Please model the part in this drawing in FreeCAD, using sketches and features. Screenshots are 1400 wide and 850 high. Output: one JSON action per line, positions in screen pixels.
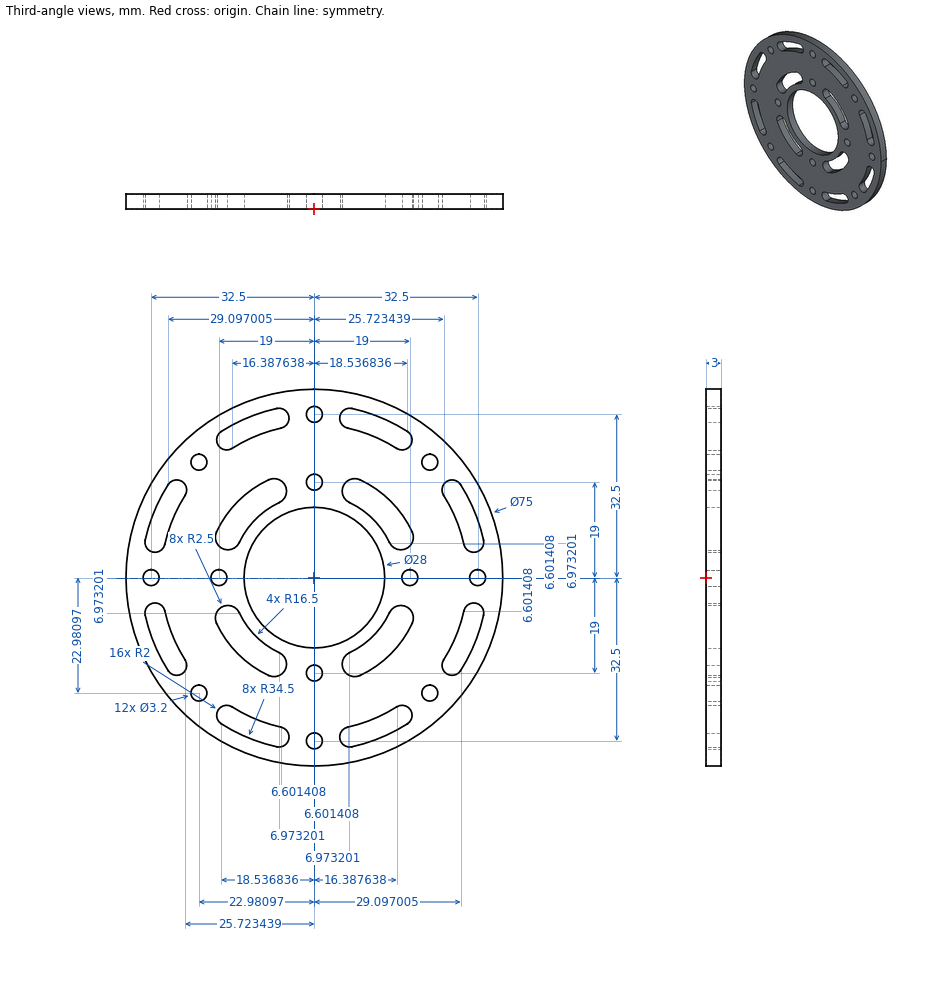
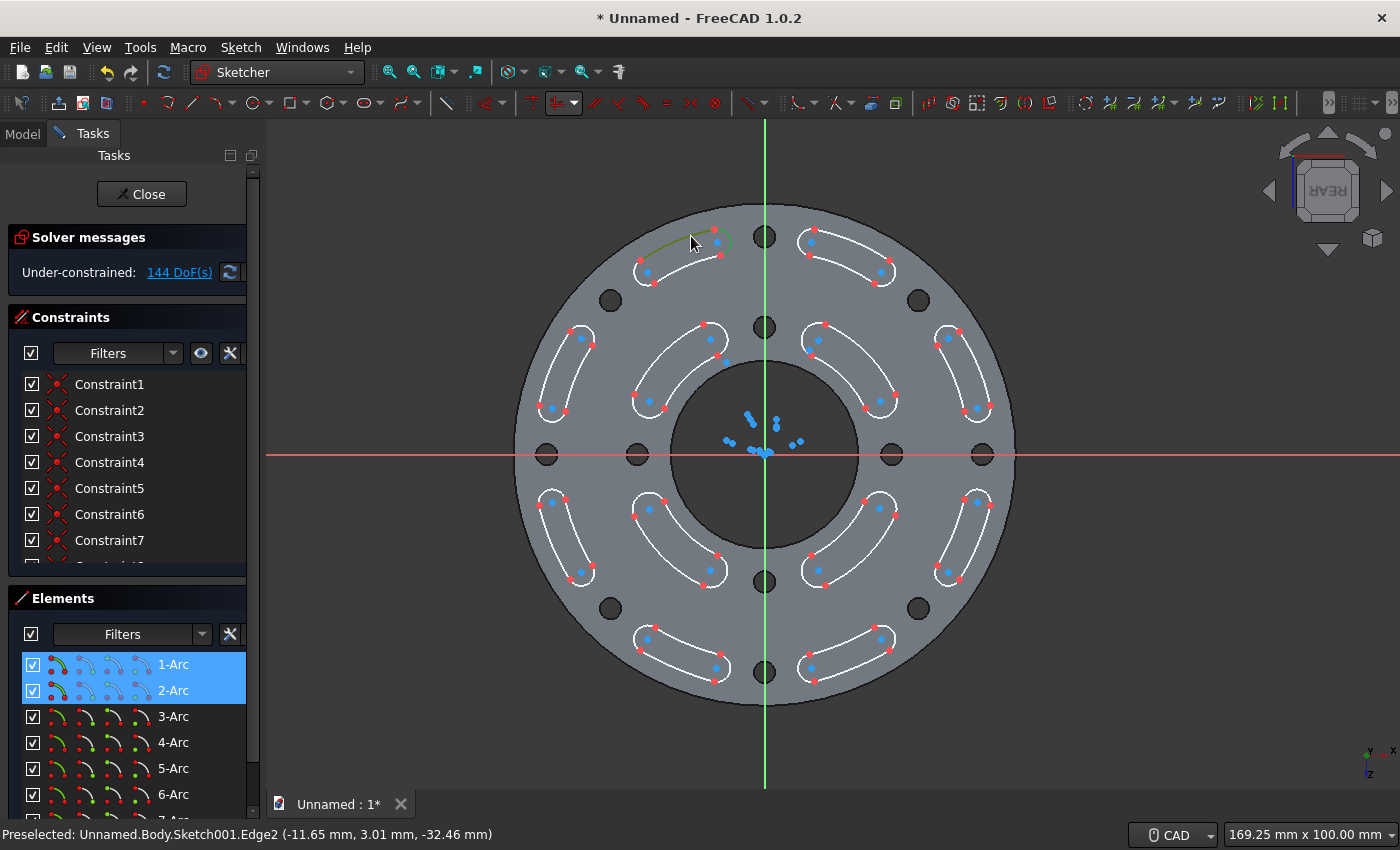
{"action": "left_click", "coordinate": [644, 104]}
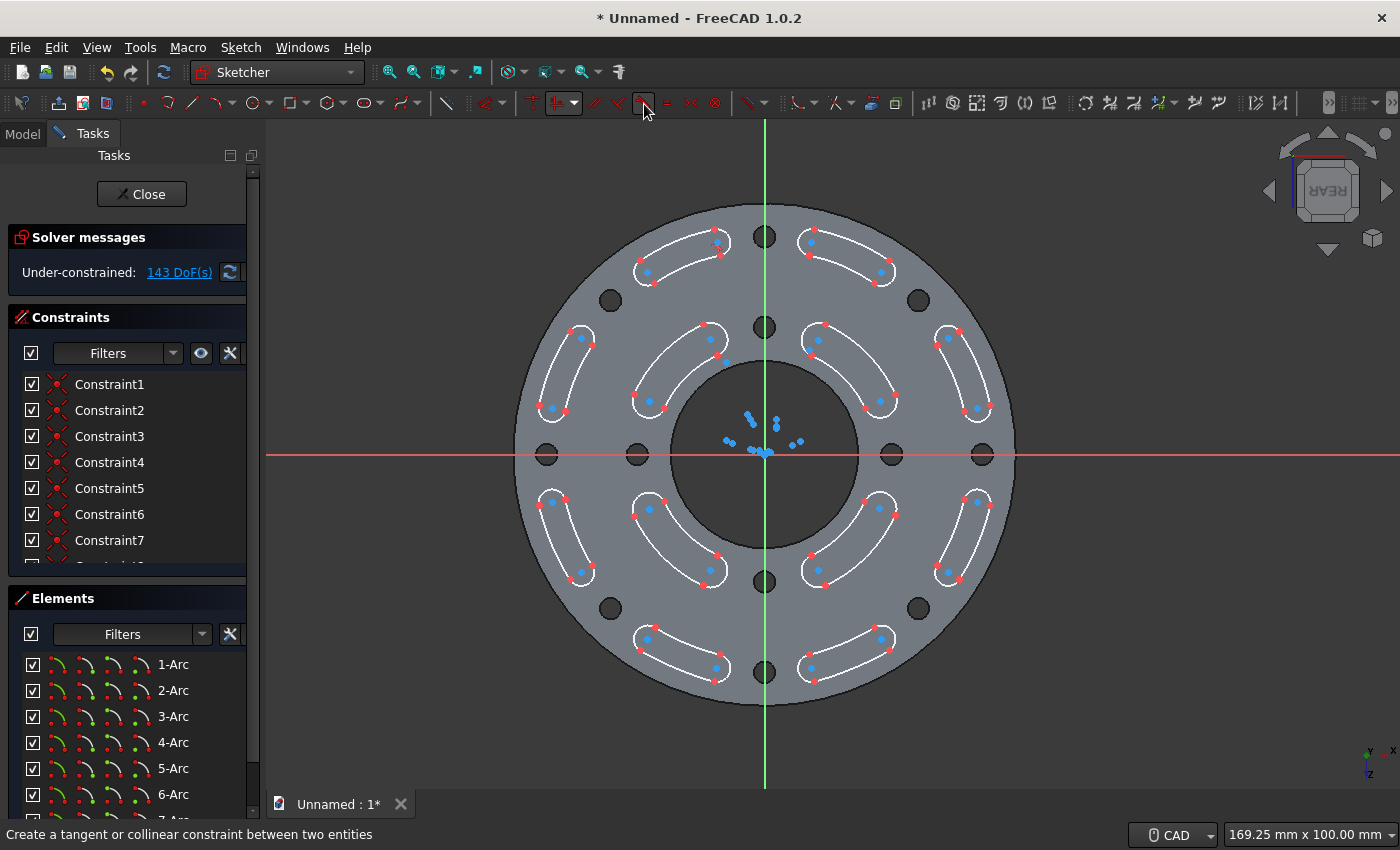
{"action": "left_click", "coordinate": [729, 248]}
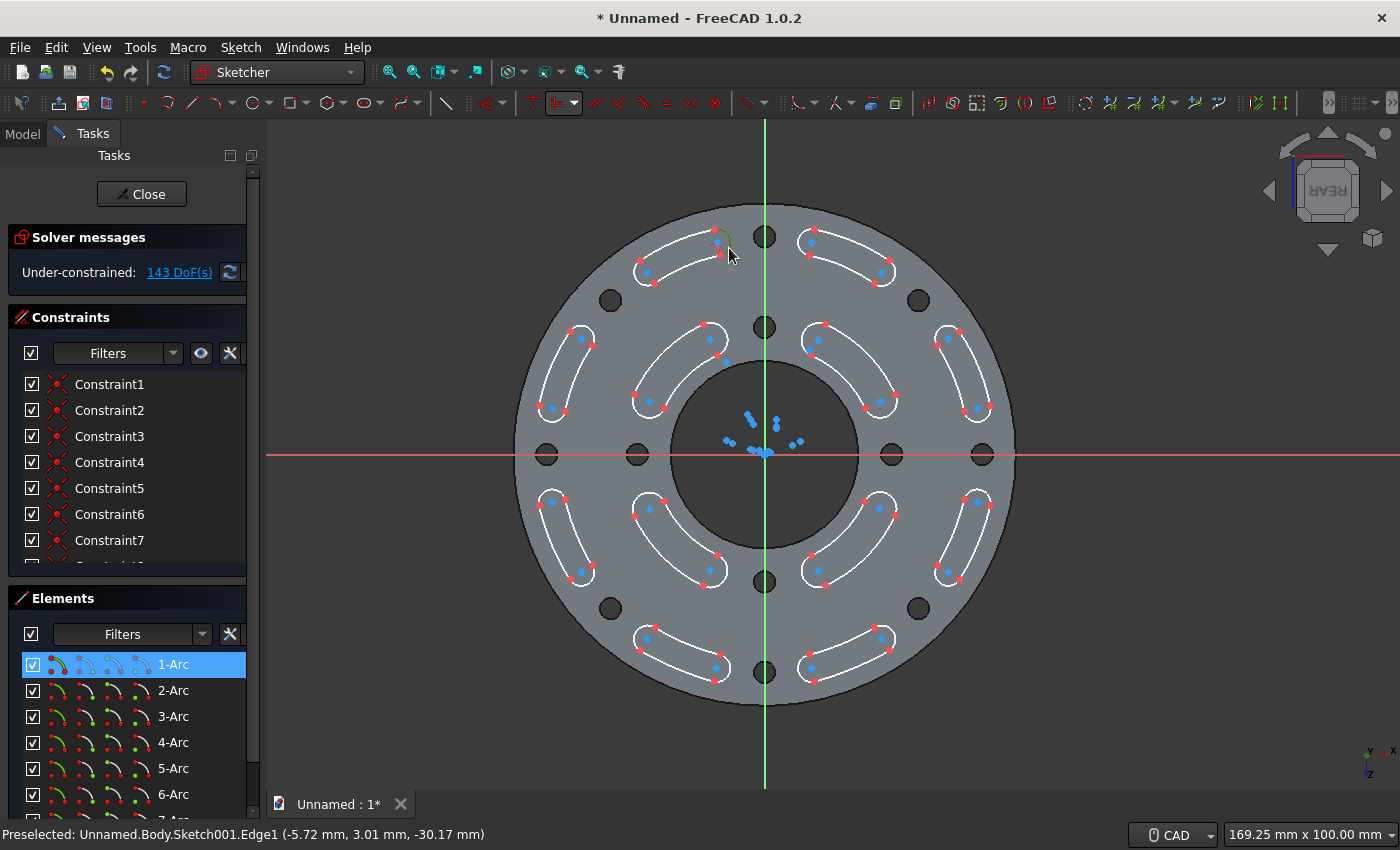
{"action": "left_click", "coordinate": [700, 261]}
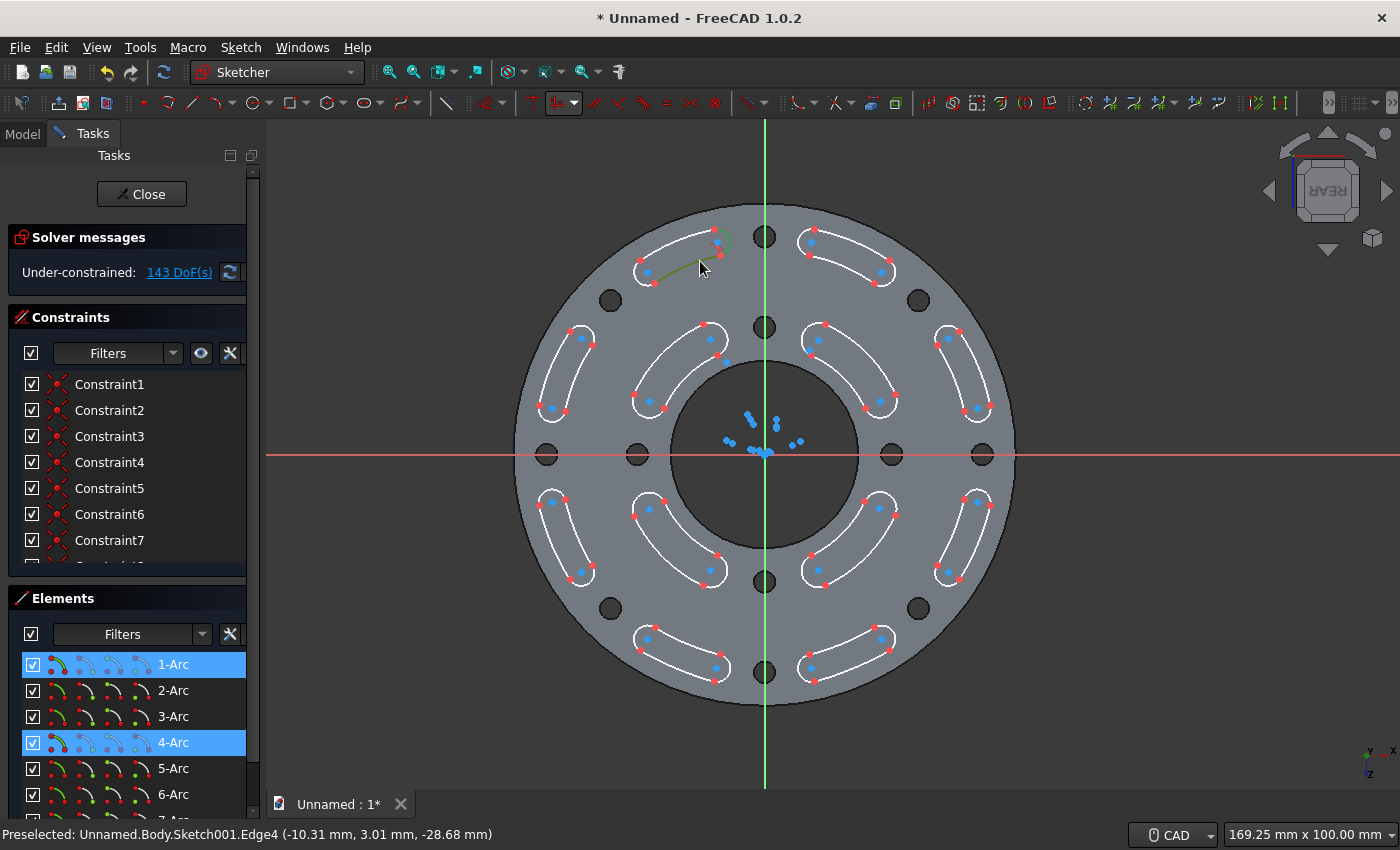
{"action": "left_click", "coordinate": [644, 104]}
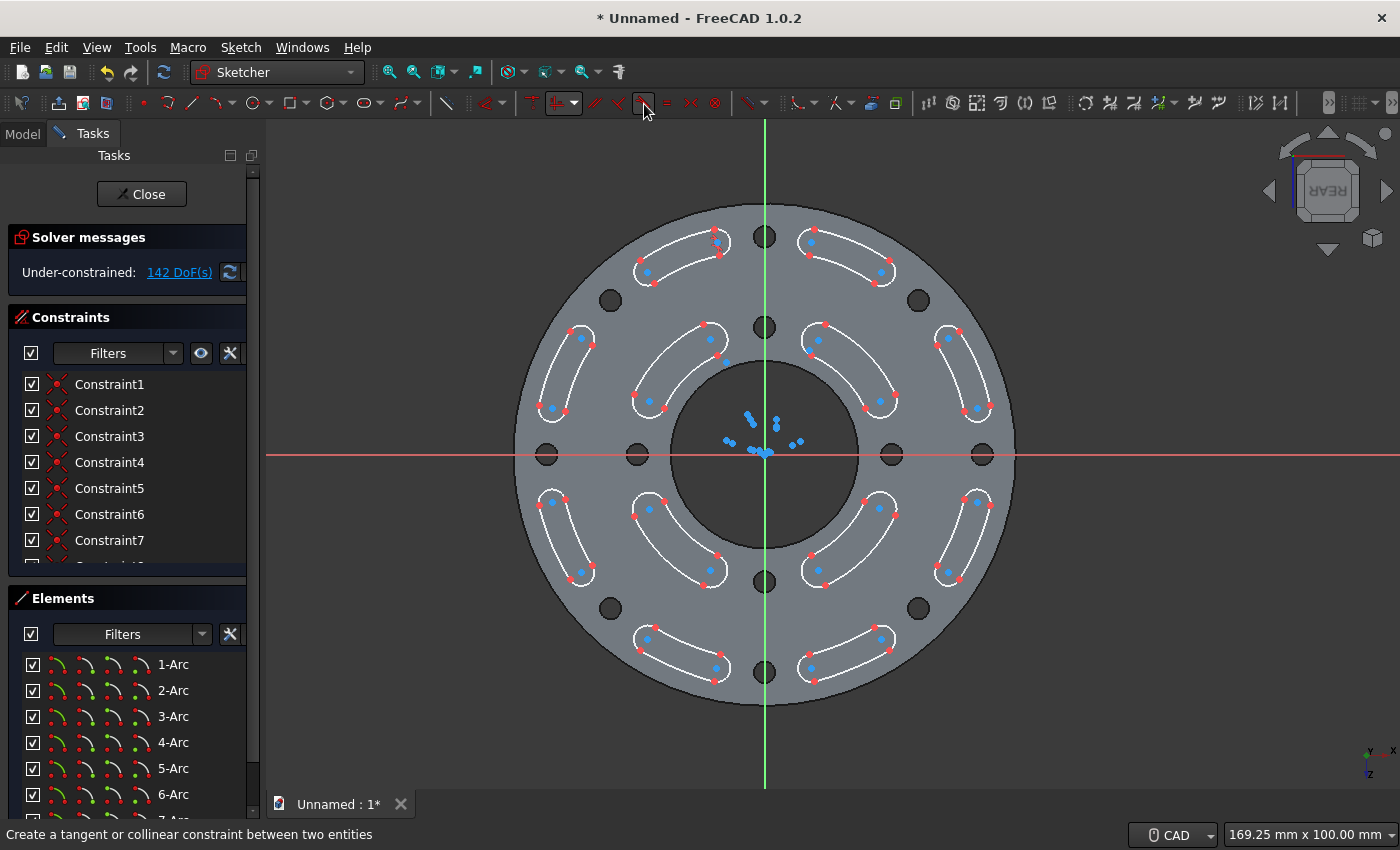
{"action": "left_click", "coordinate": [691, 236]}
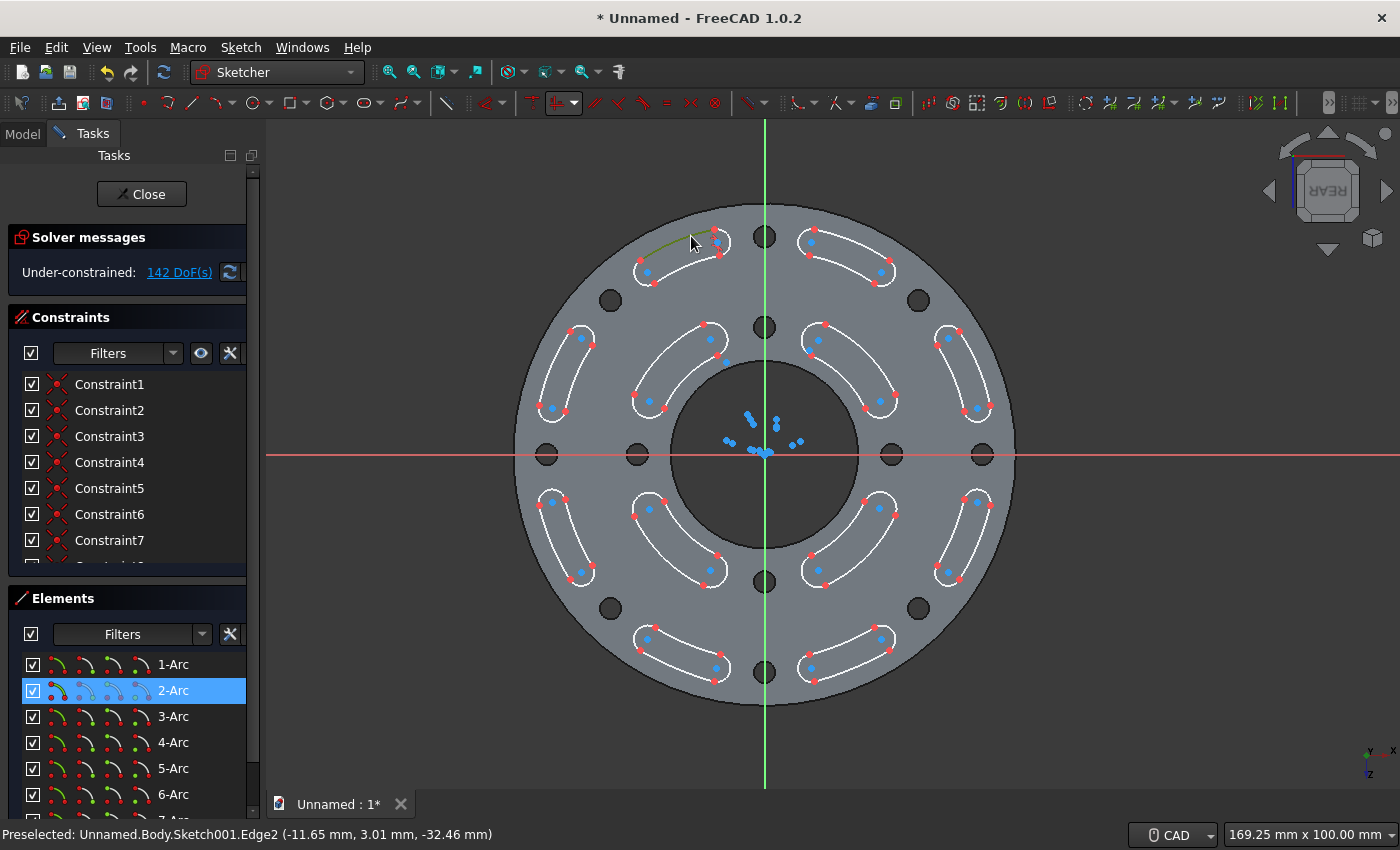
{"action": "left_click", "coordinate": [634, 271]}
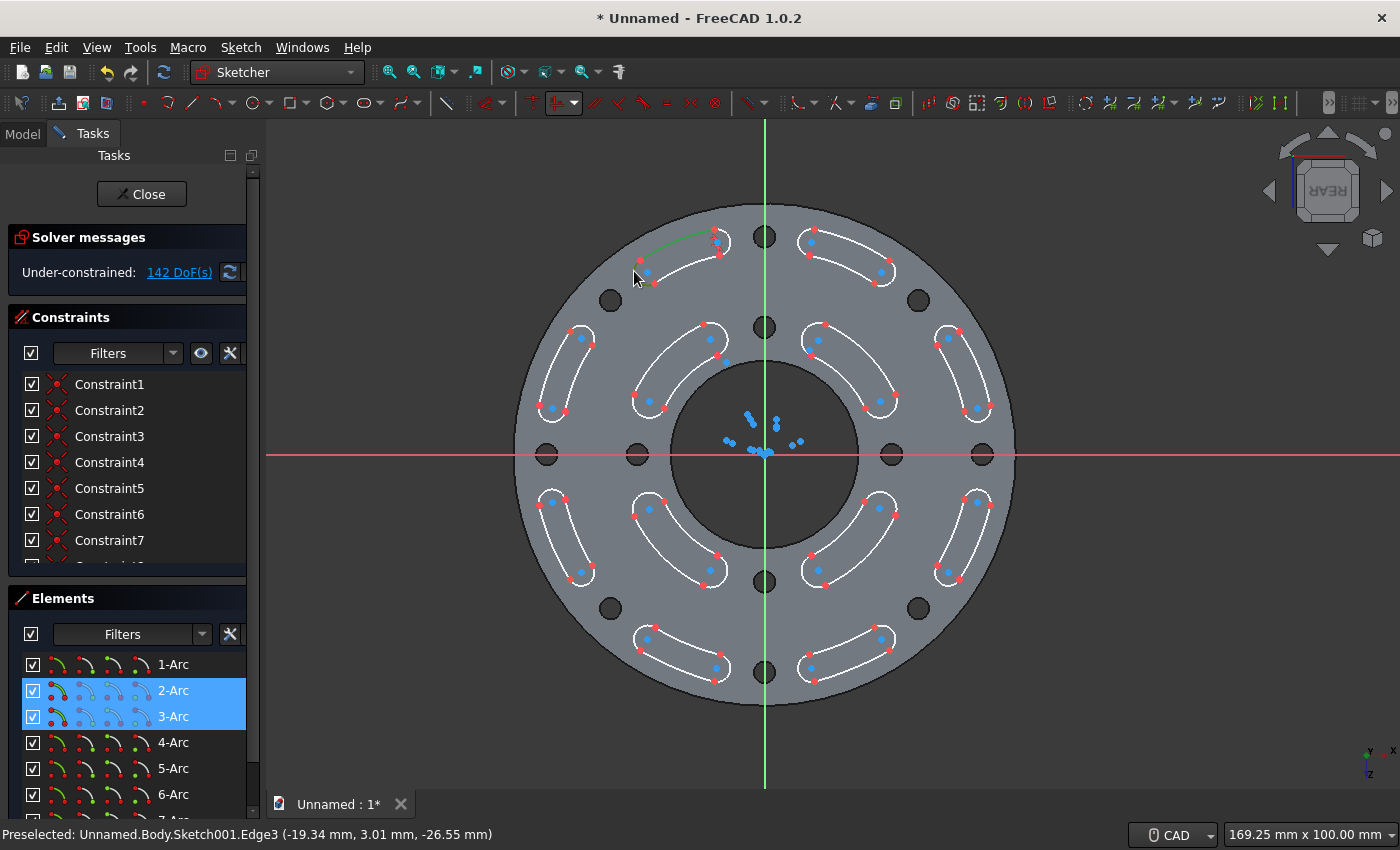
{"action": "left_click", "coordinate": [644, 104]}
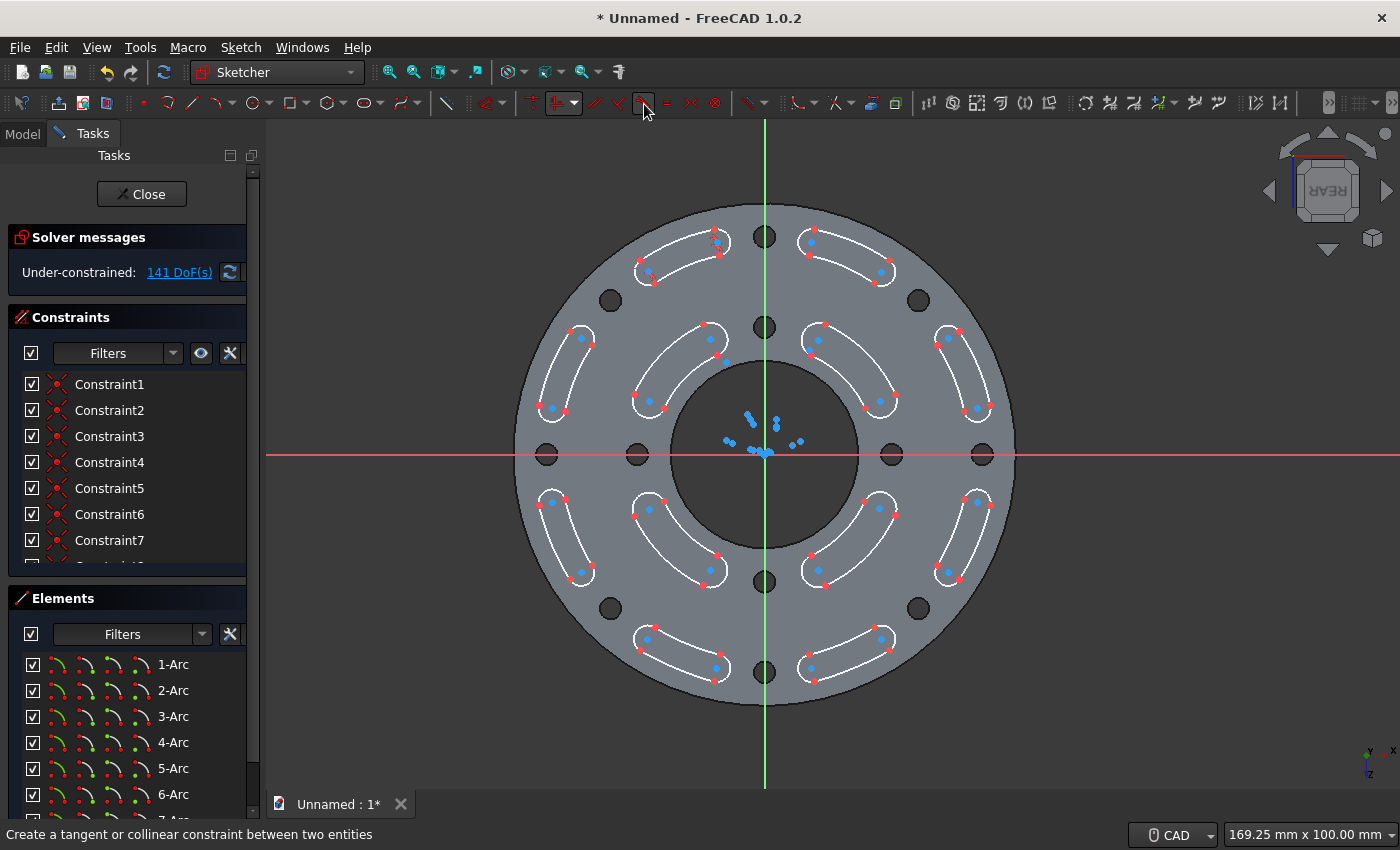
{"action": "left_click", "coordinate": [635, 271]}